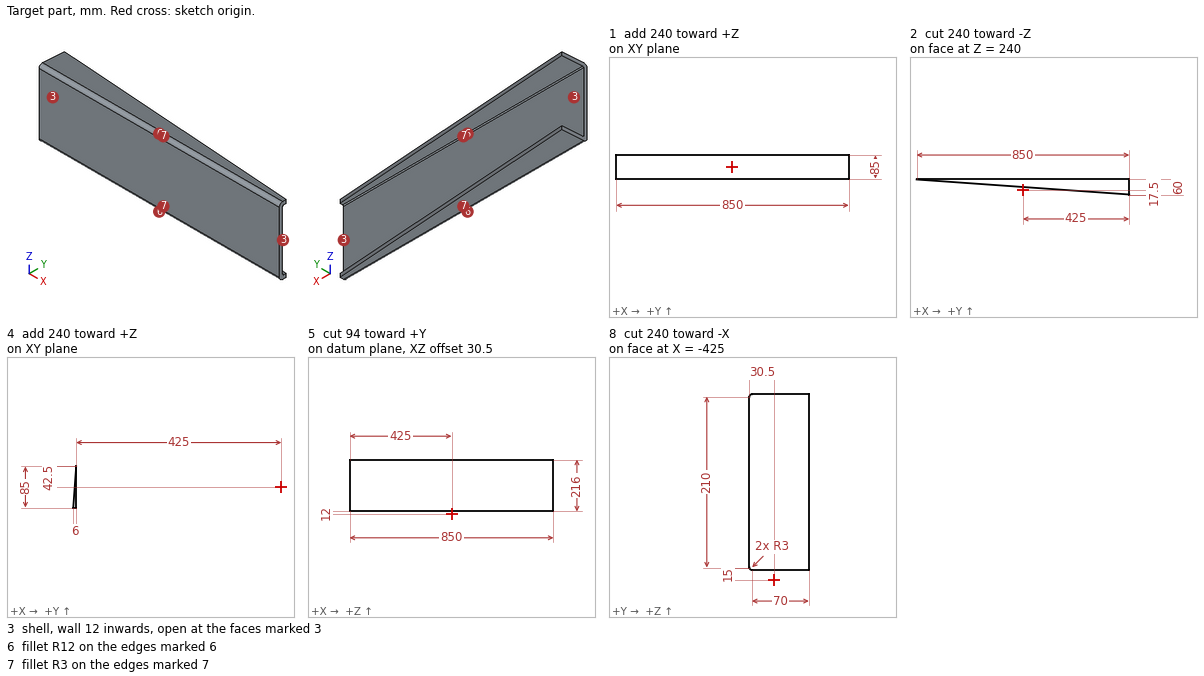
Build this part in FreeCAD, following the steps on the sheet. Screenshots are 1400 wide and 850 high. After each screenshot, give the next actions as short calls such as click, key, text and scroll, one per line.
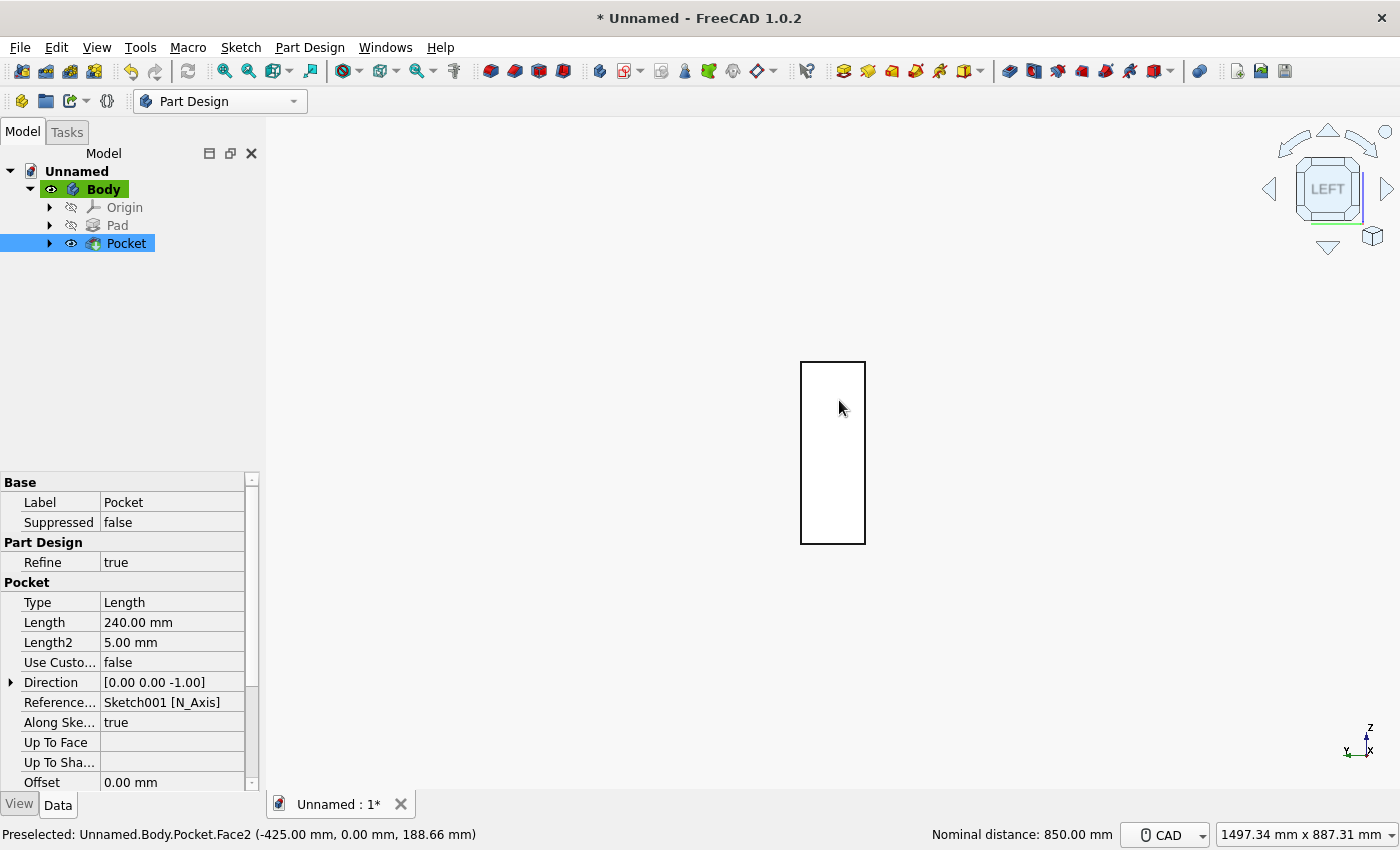
click(564, 72)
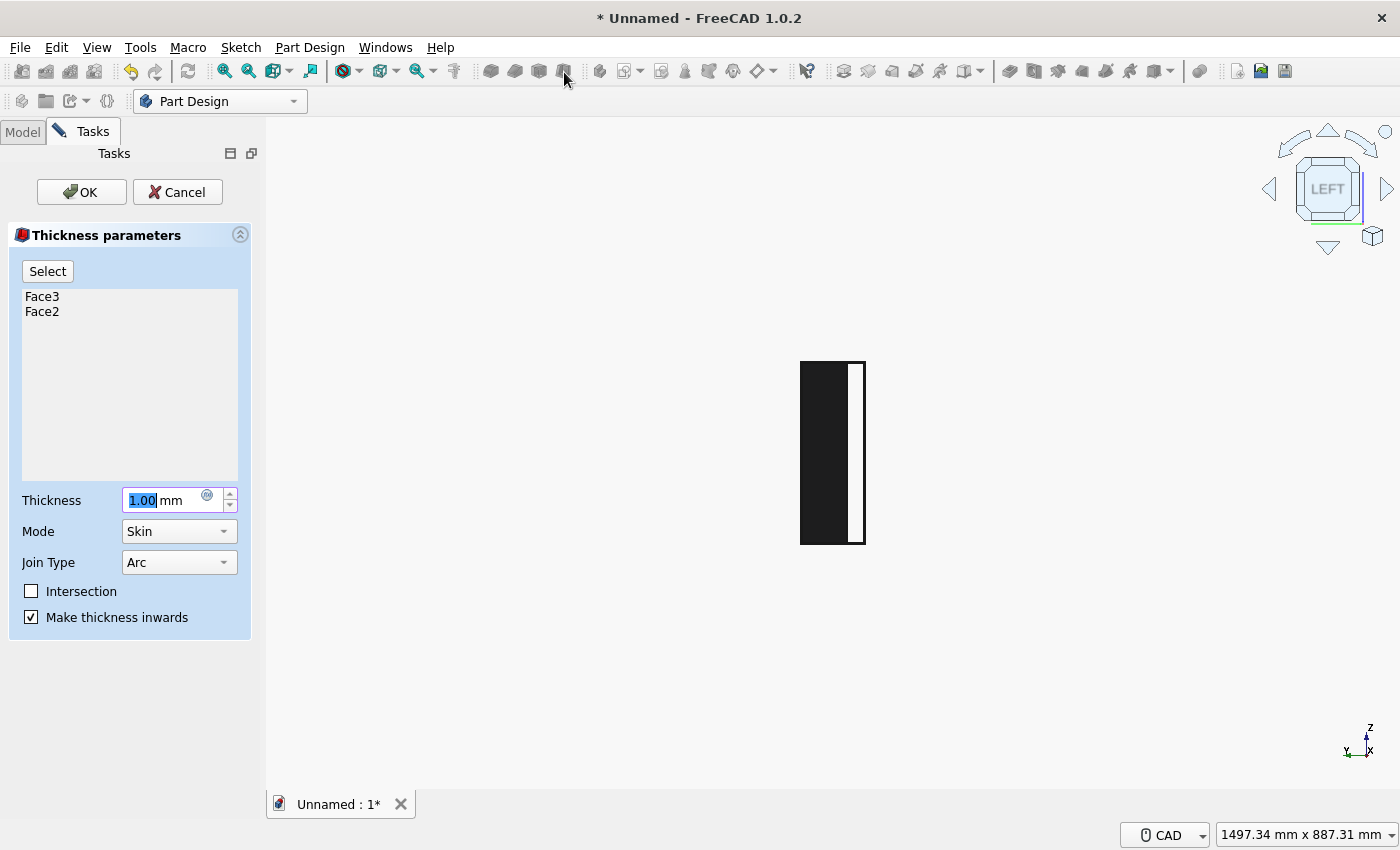
text(12)
key(Tab)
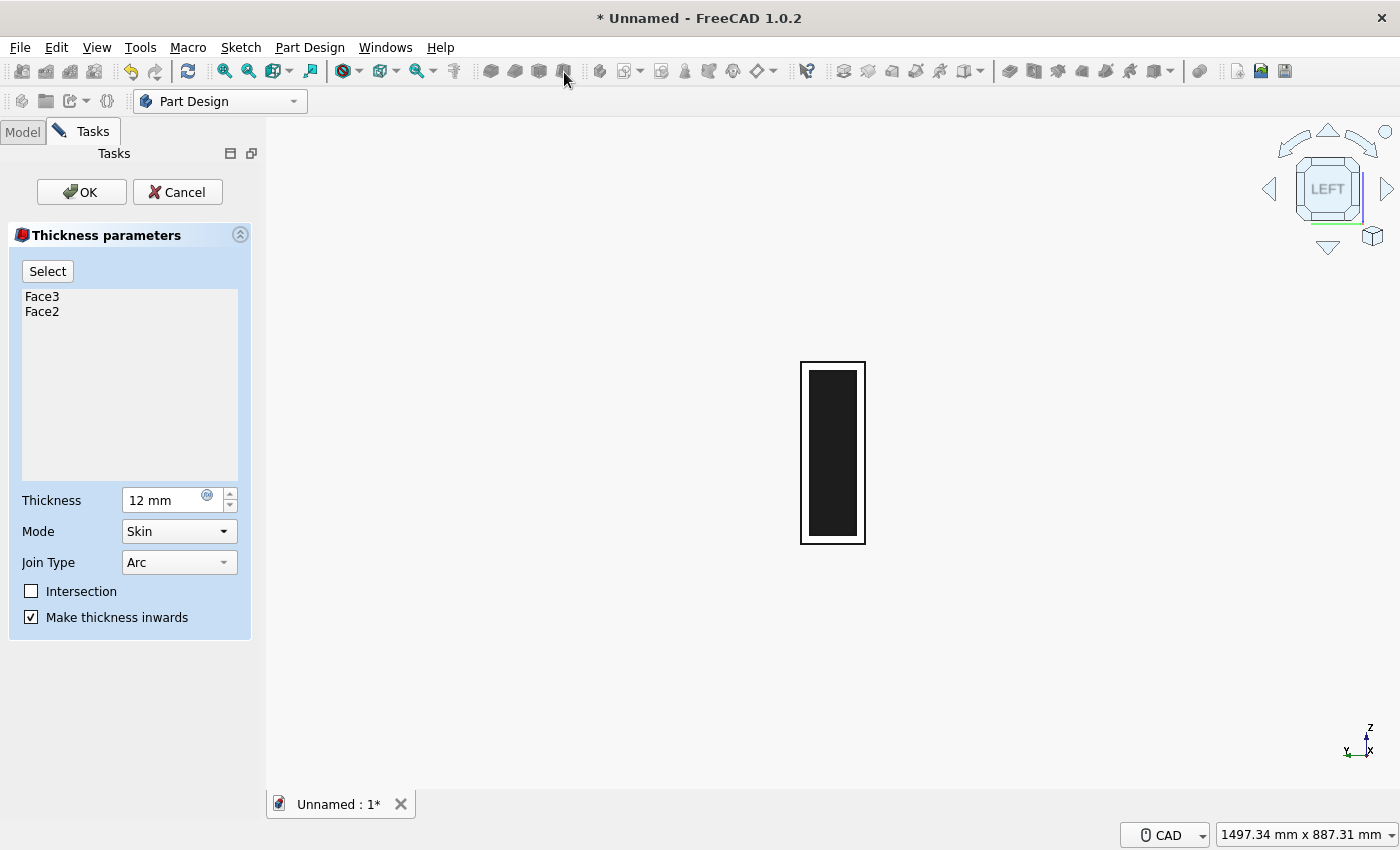
click(180, 562)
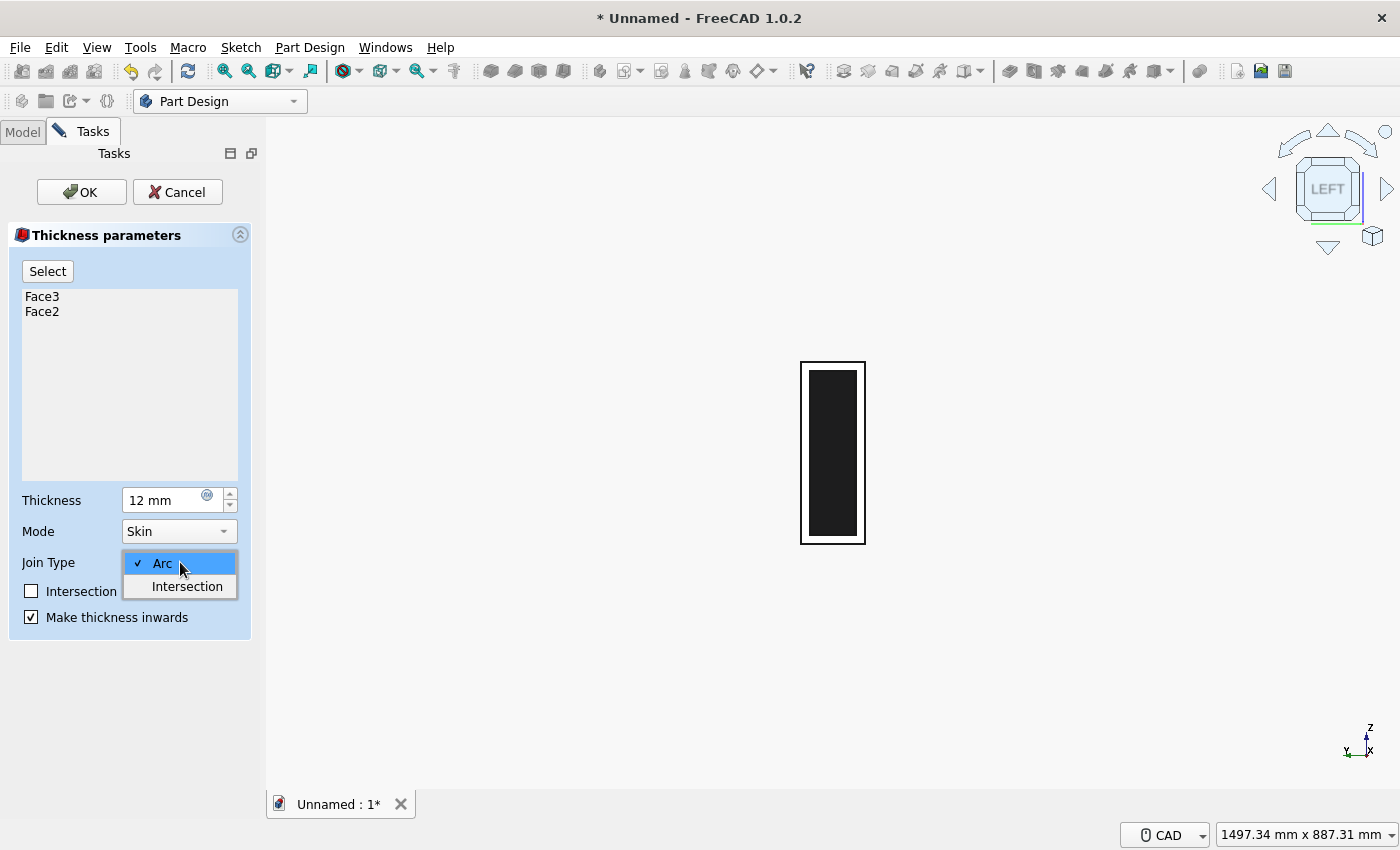
click(179, 586)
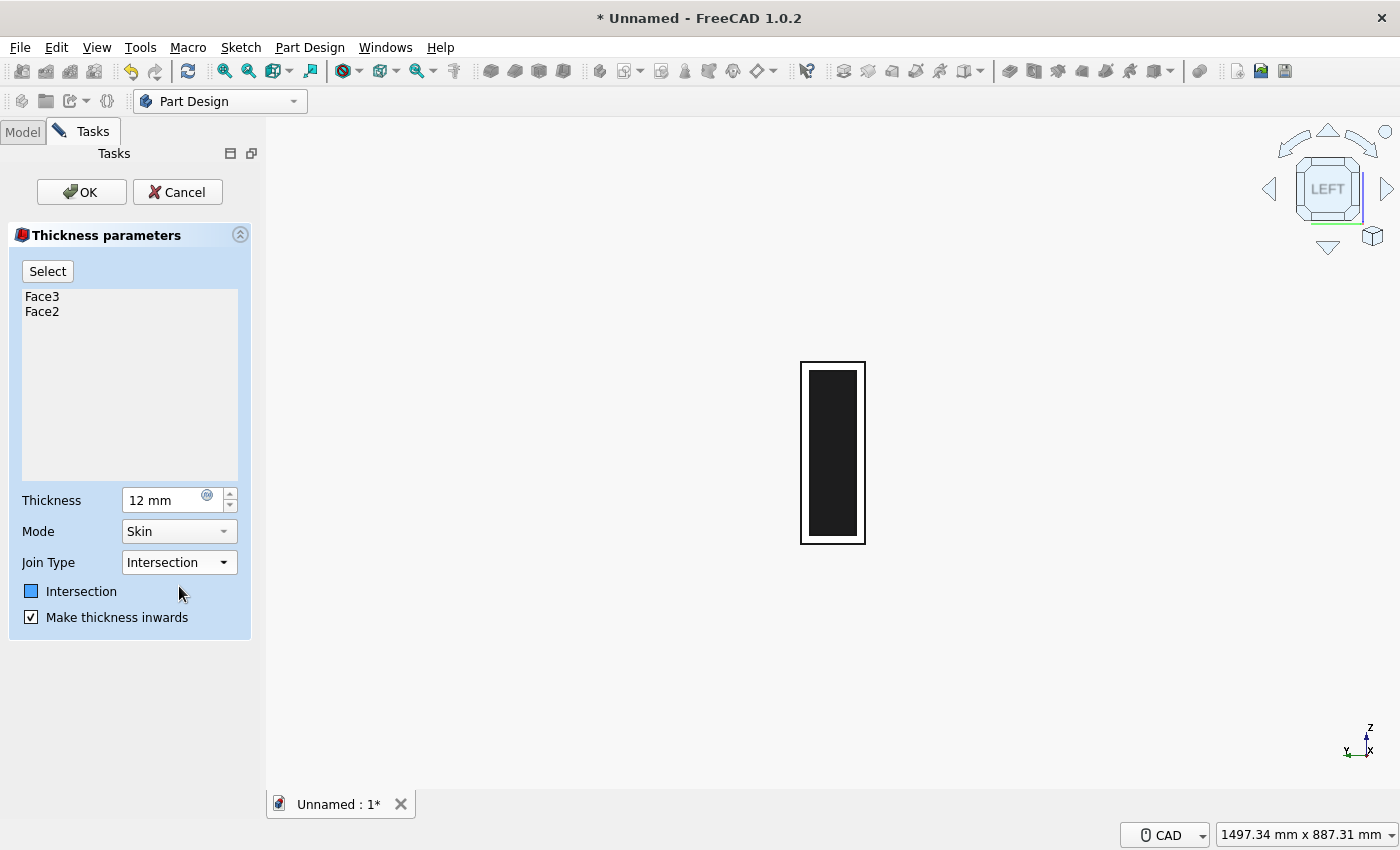
click(82, 192)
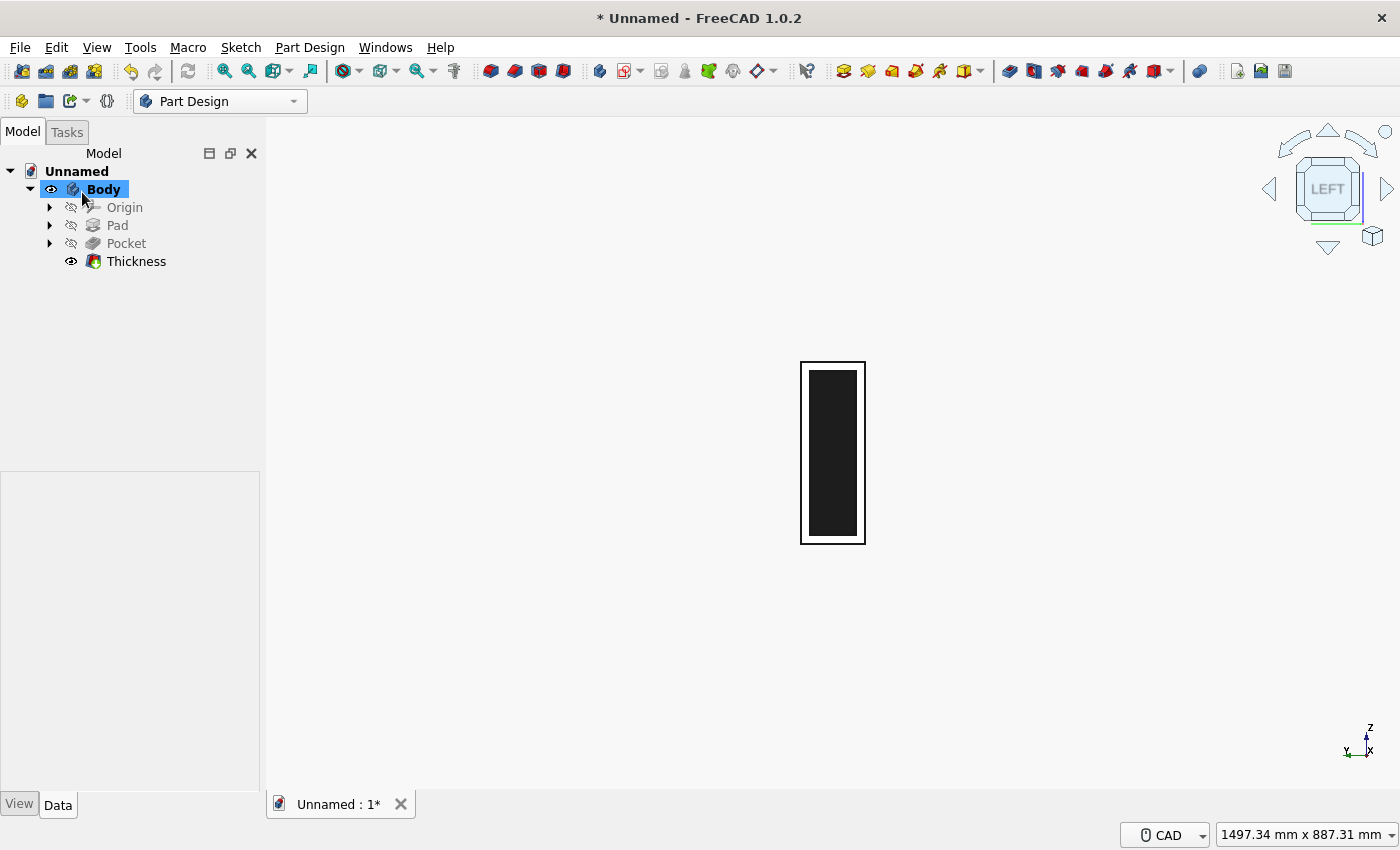
key(v)
key(f)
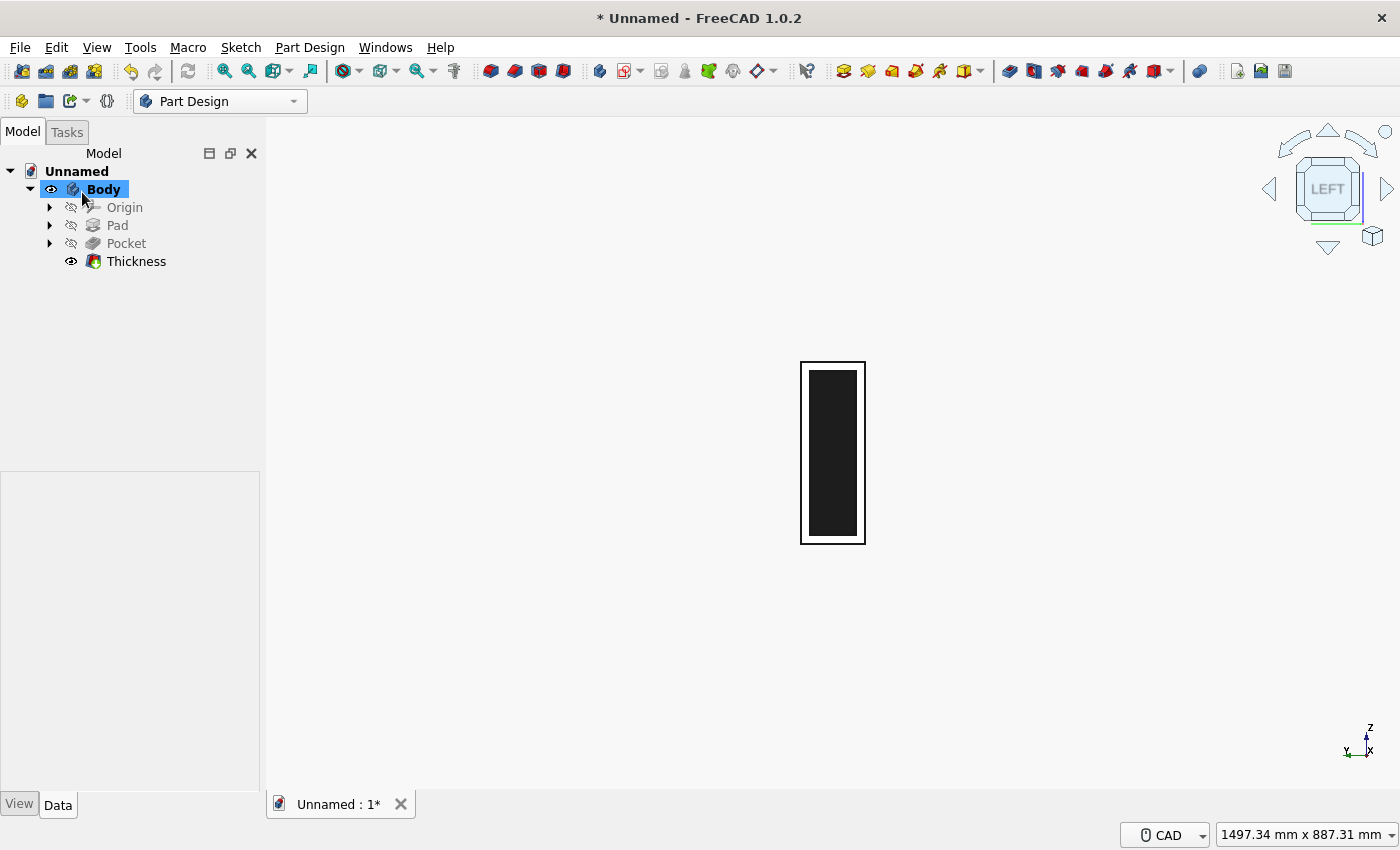
click(624, 72)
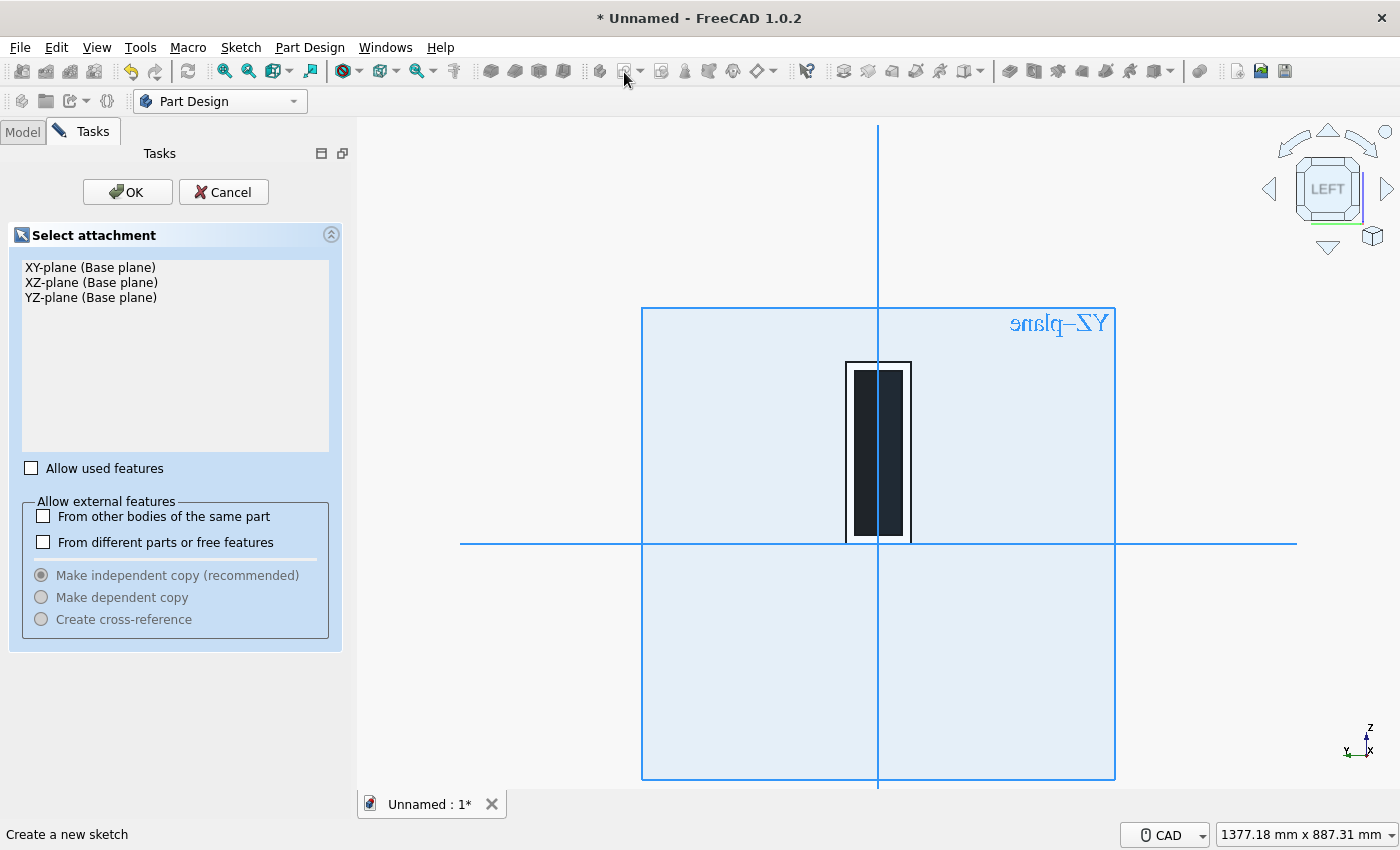
click(82, 268)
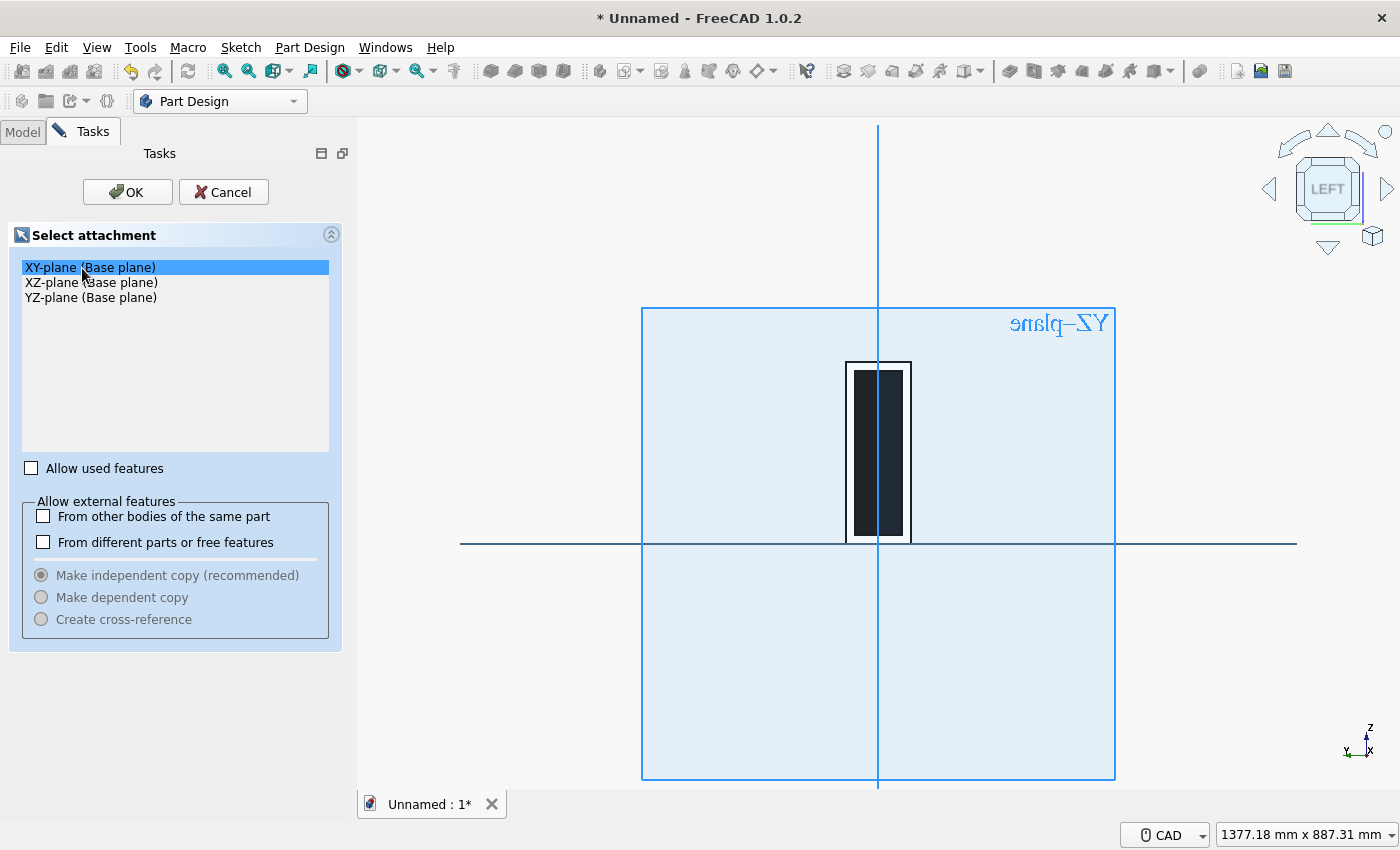
click(128, 192)